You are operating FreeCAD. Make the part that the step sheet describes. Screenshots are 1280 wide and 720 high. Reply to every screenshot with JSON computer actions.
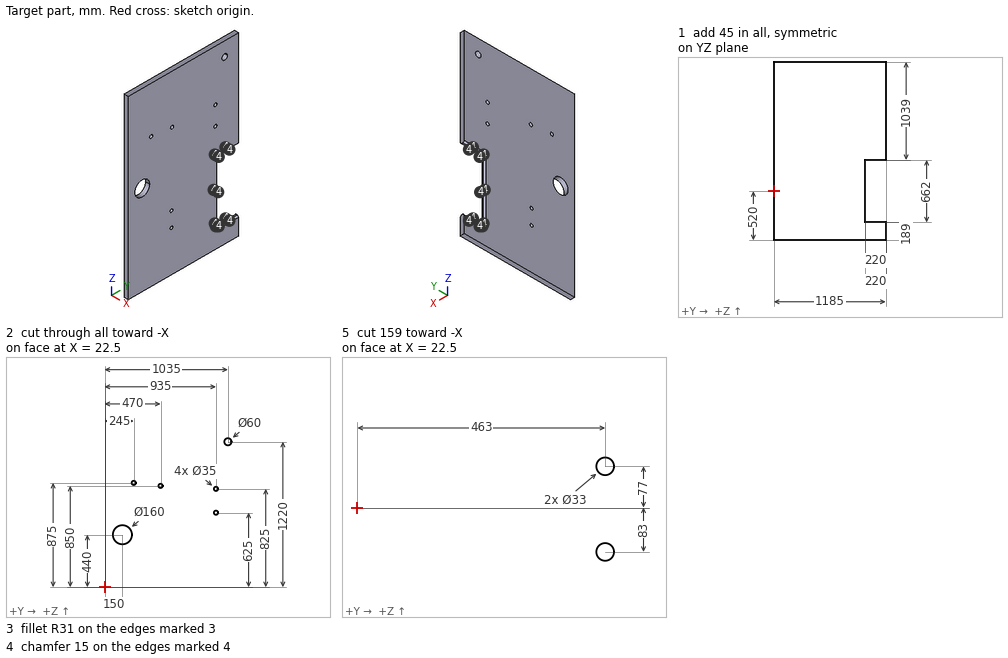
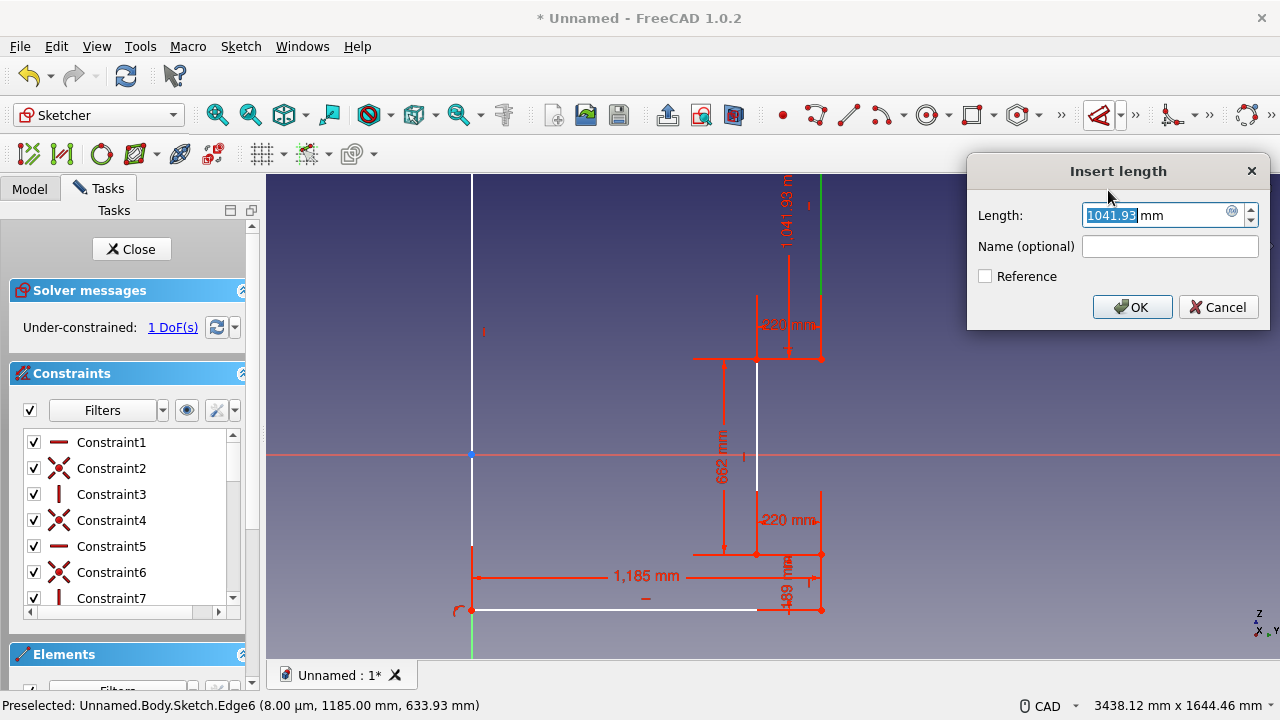
{"action": "type", "text": "1039"}
{"action": "key", "text": "Return"}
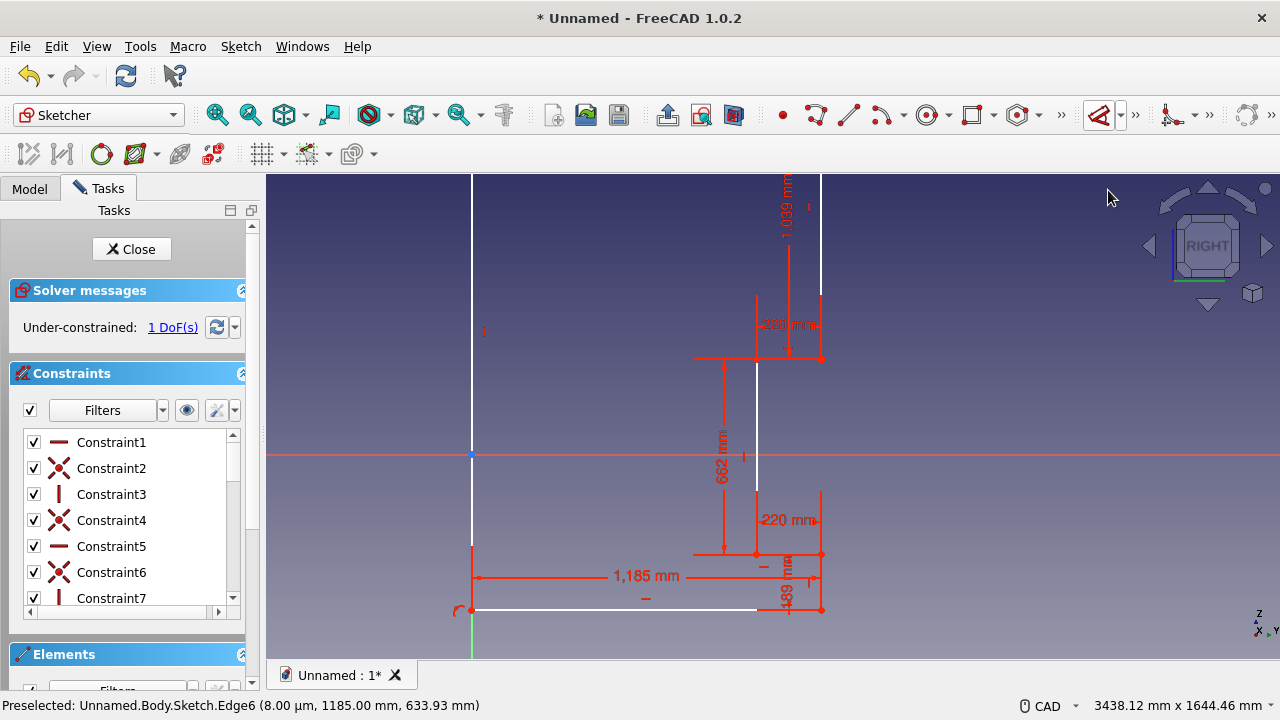
{"action": "left_click", "coordinate": [472, 610]}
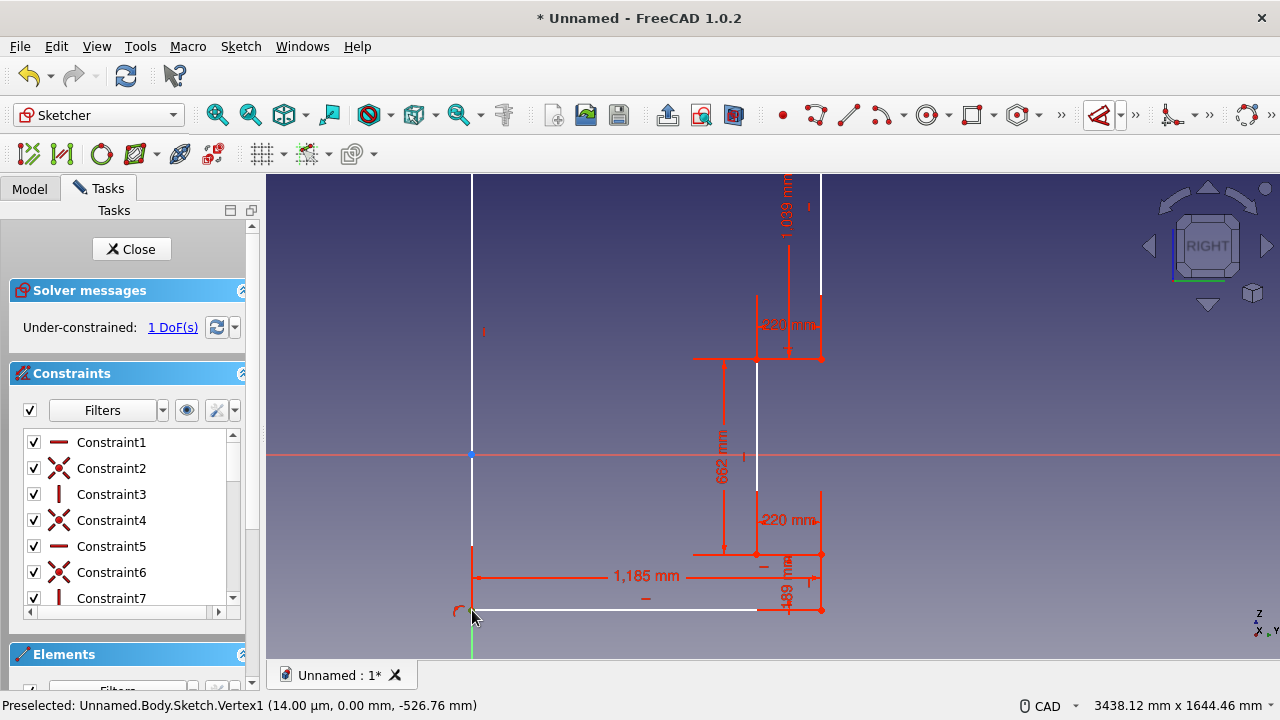
{"action": "key", "text": "i"}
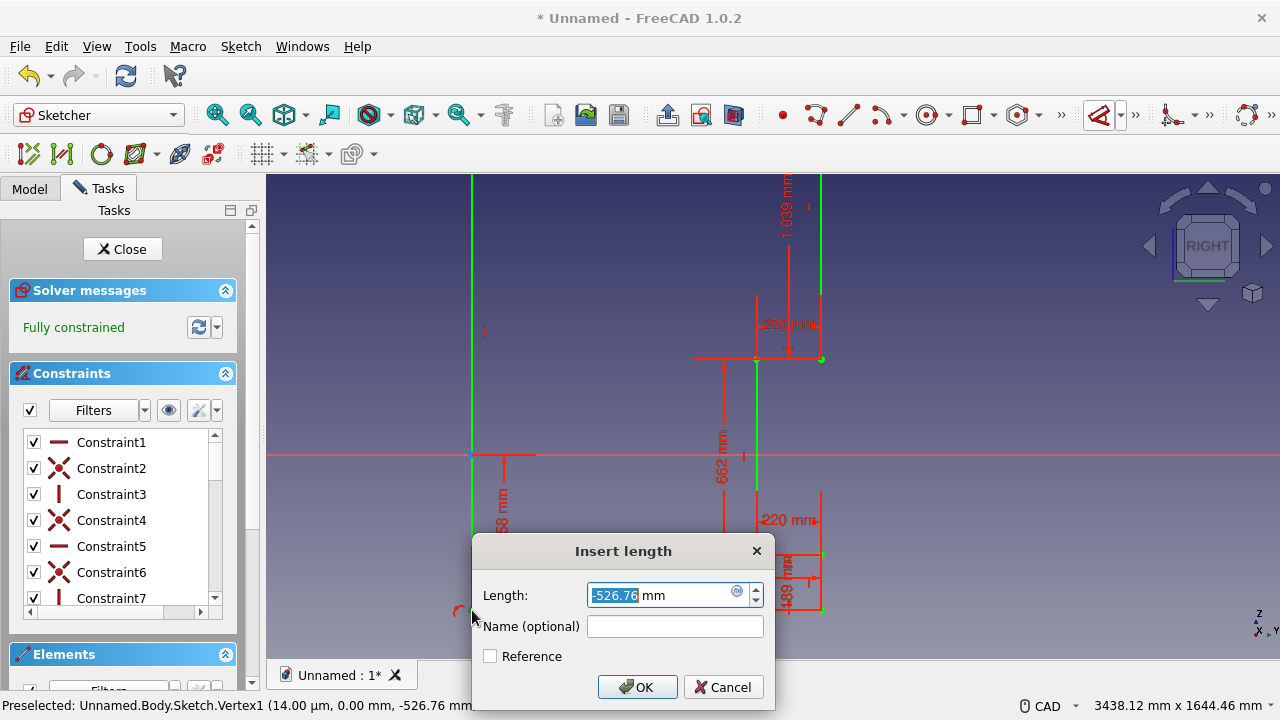
{"action": "type", "text": "-520"}
{"action": "key", "text": "Return"}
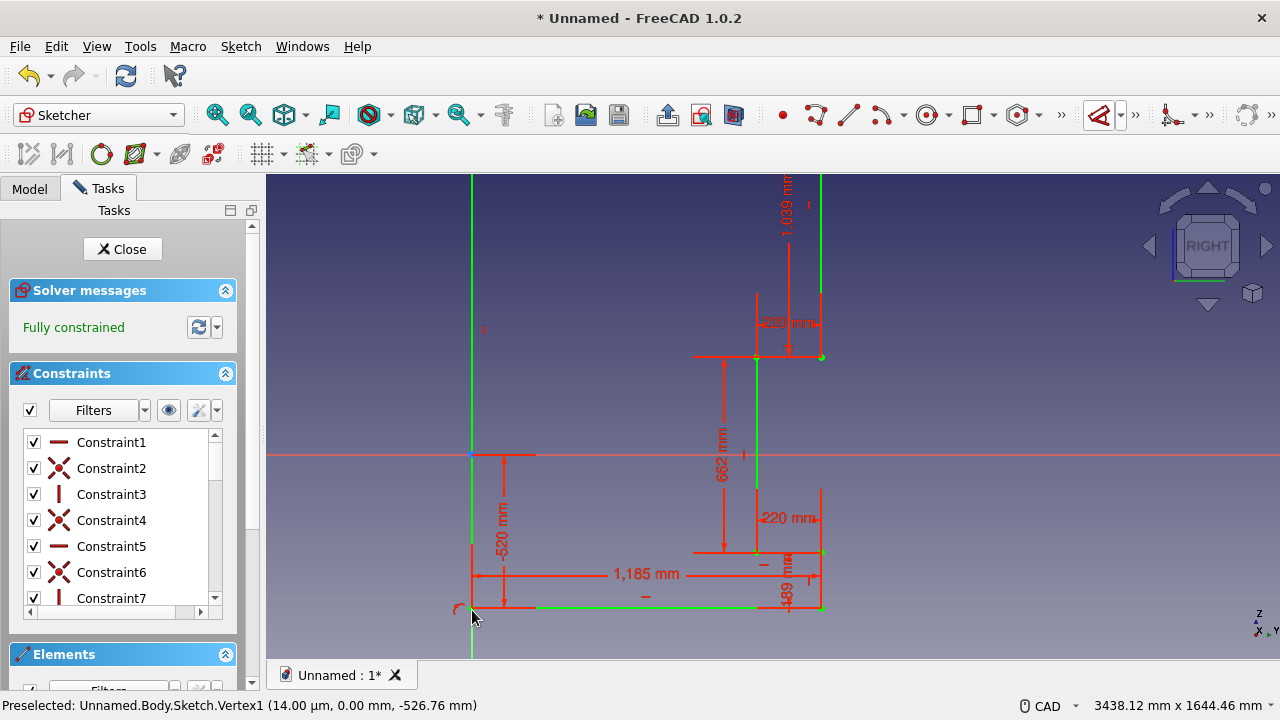
{"action": "left_click", "coordinate": [123, 249]}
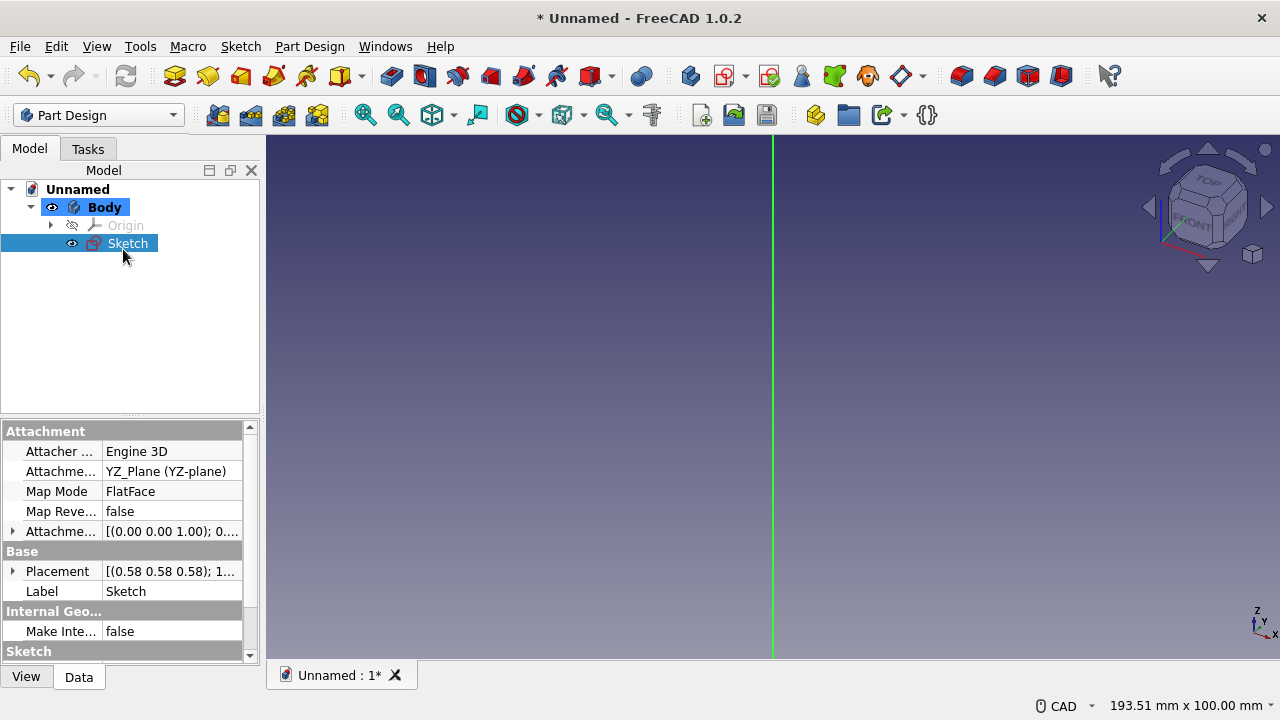
{"action": "left_click", "coordinate": [175, 76]}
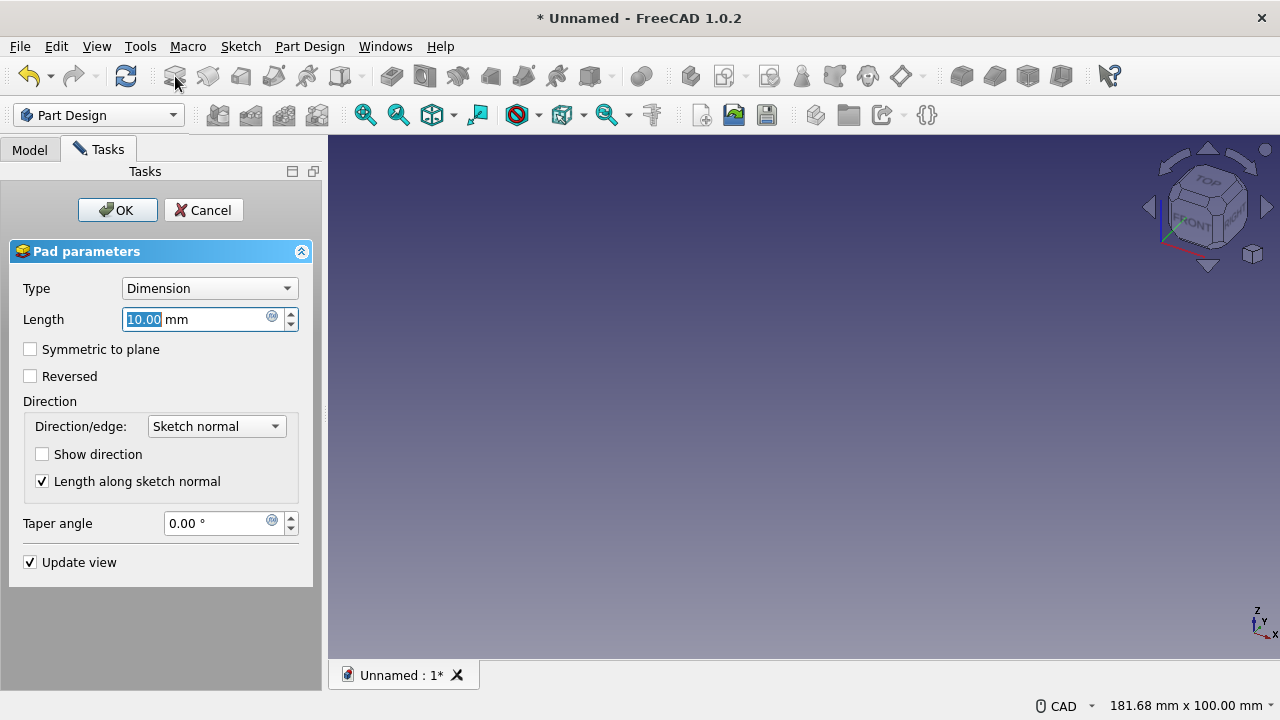
{"action": "type", "text": "45"}
{"action": "key", "text": "Tab"}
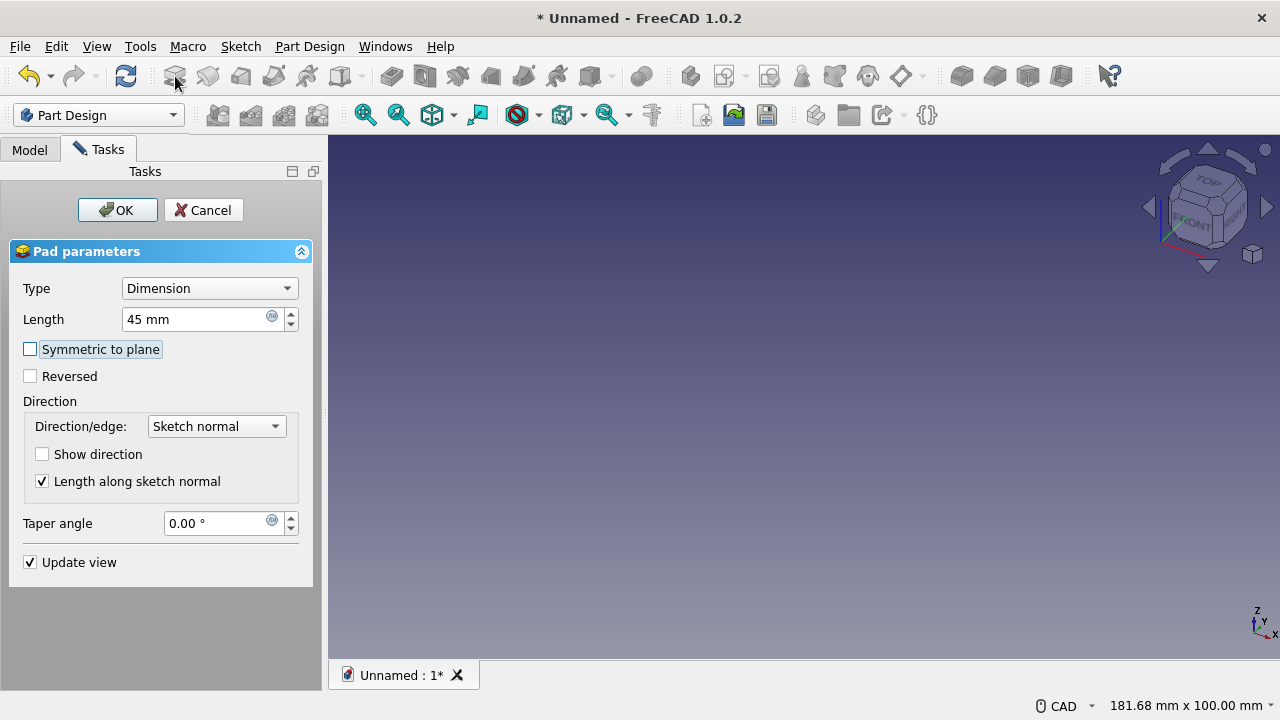
{"action": "left_click", "coordinate": [31, 349]}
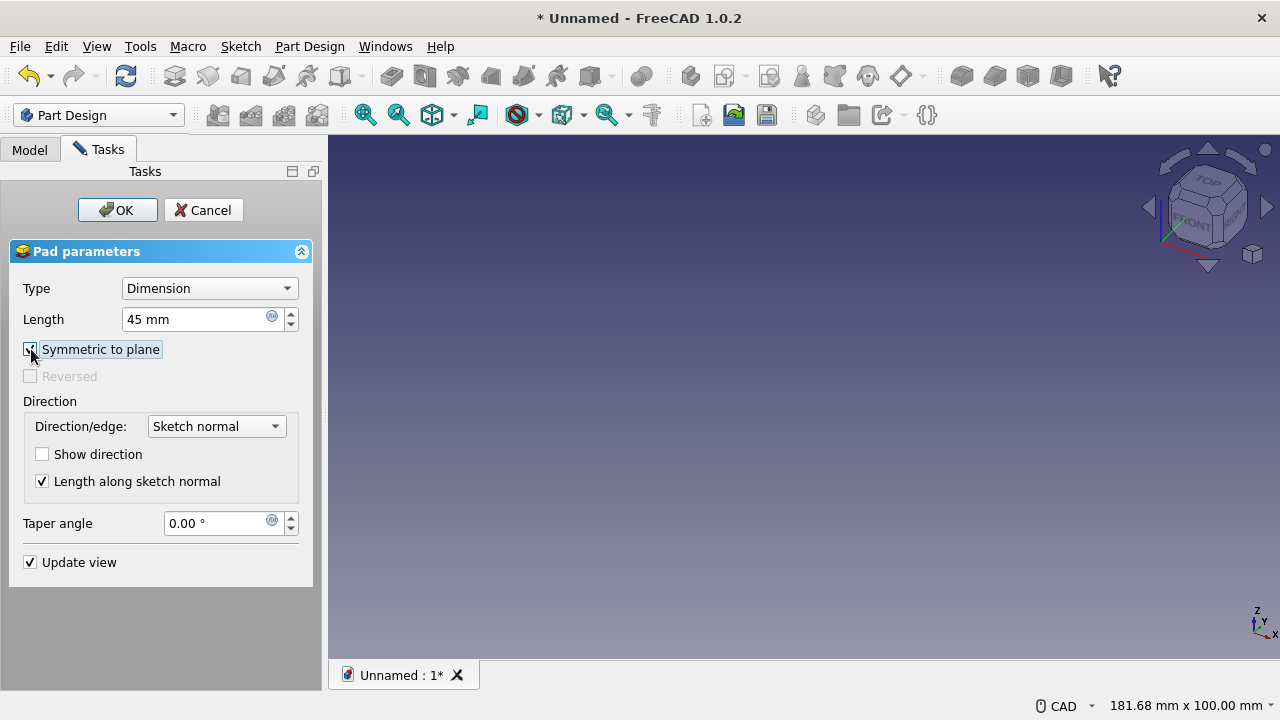
{"action": "left_click", "coordinate": [118, 210]}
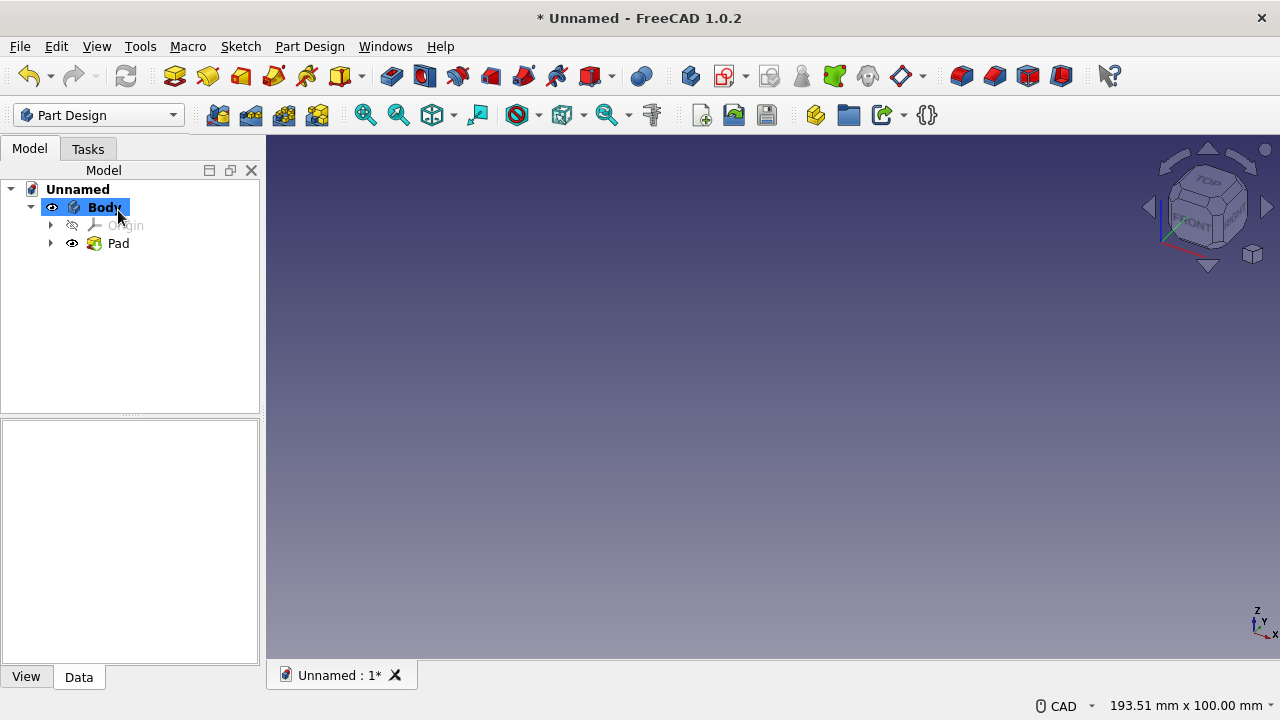
{"action": "key", "text": "v f"}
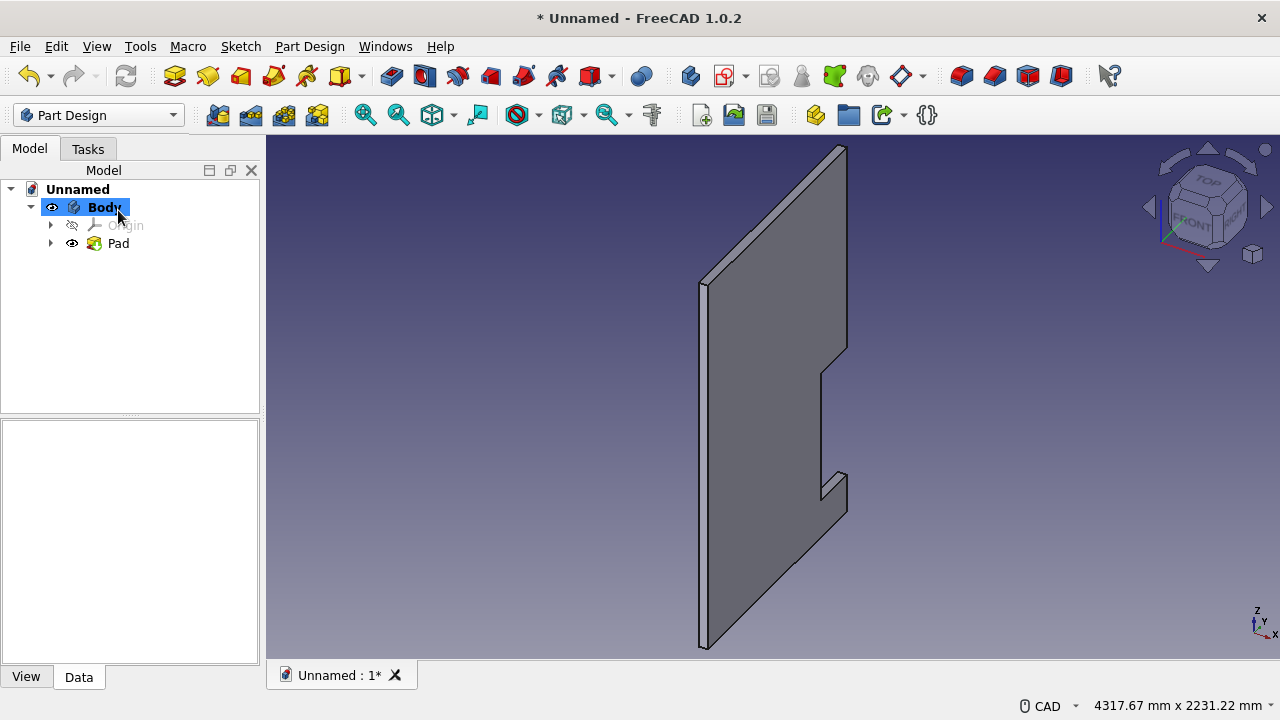
{"action": "left_click", "coordinate": [778, 346]}